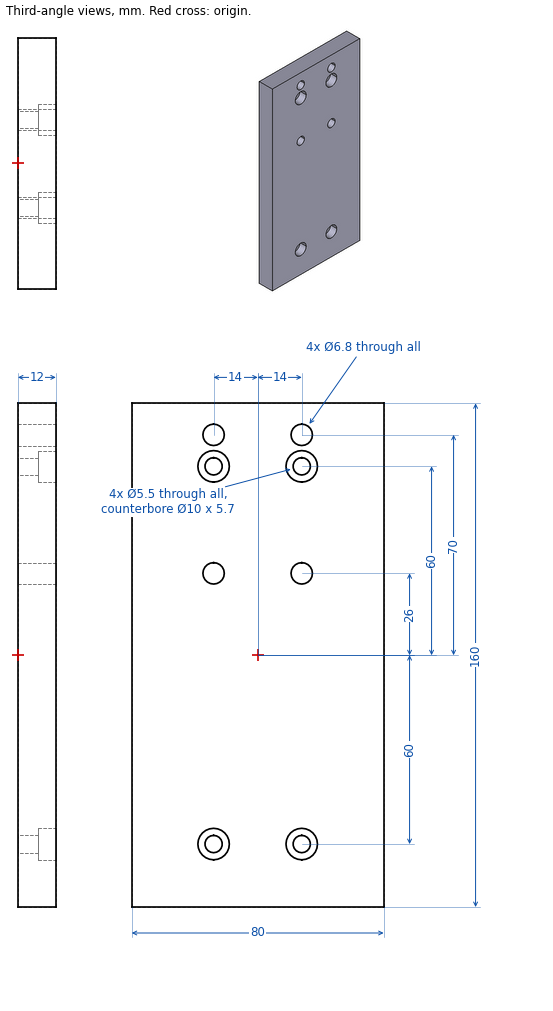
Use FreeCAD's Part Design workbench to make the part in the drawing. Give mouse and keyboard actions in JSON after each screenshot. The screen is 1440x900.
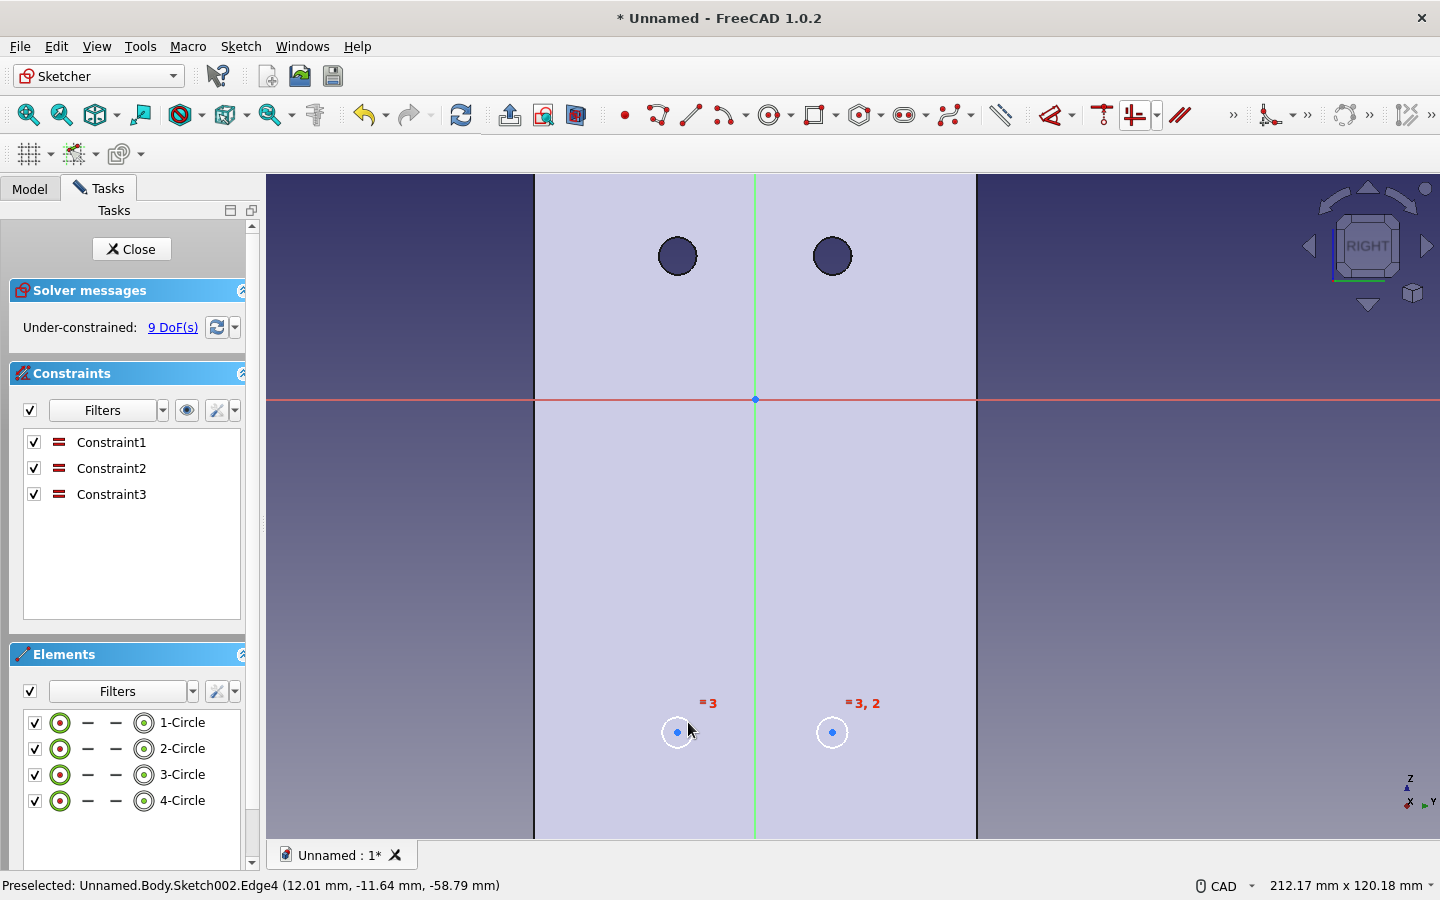
{"action": "scroll", "coordinate": [844, 723], "scroll_direction": "down", "scroll_amount": 2}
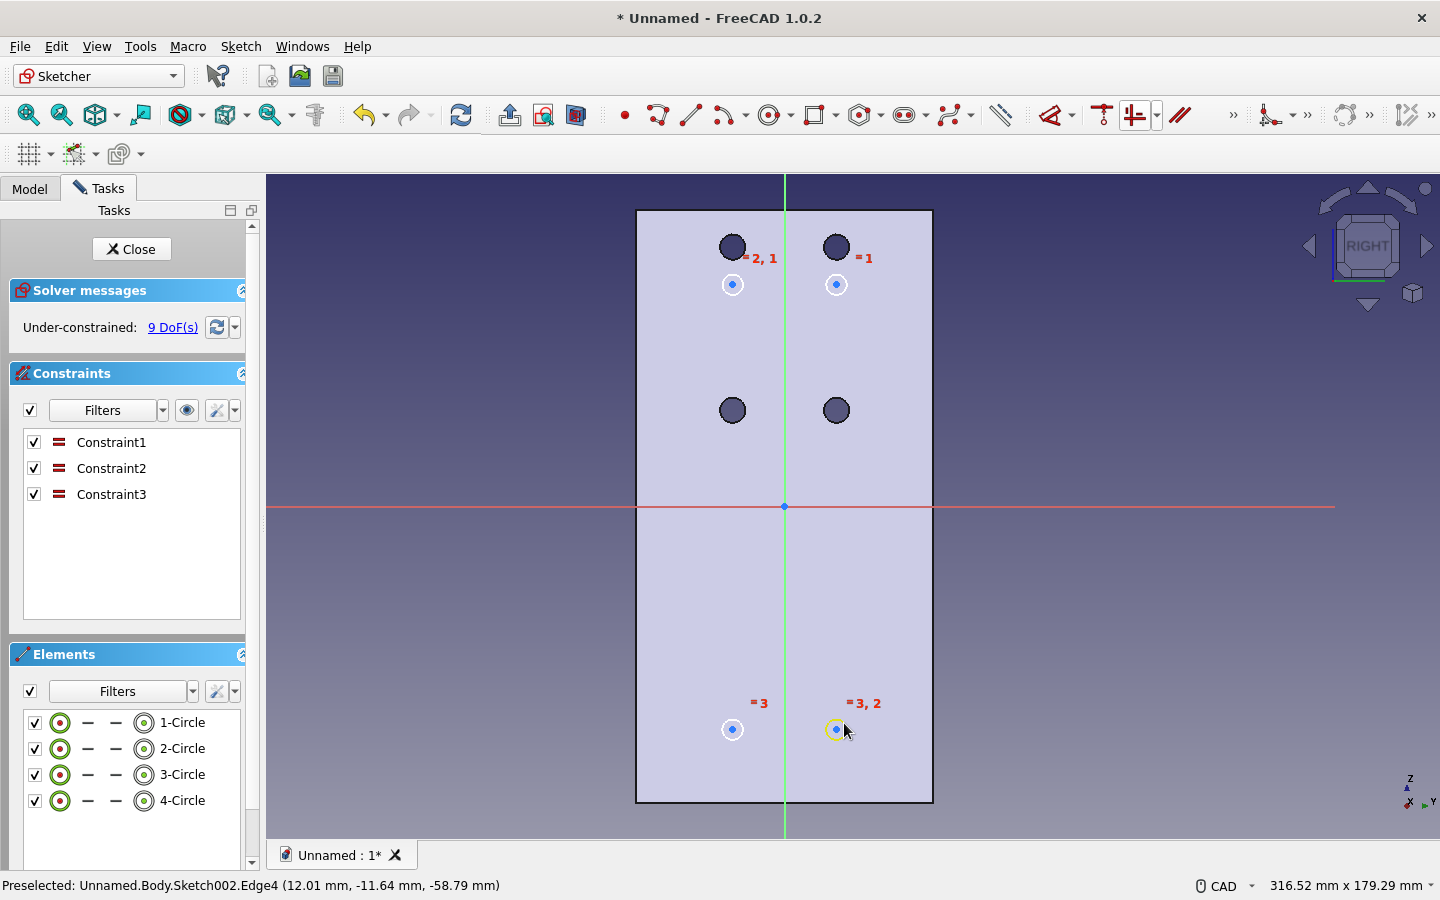
{"action": "left_click", "coordinate": [837, 285]}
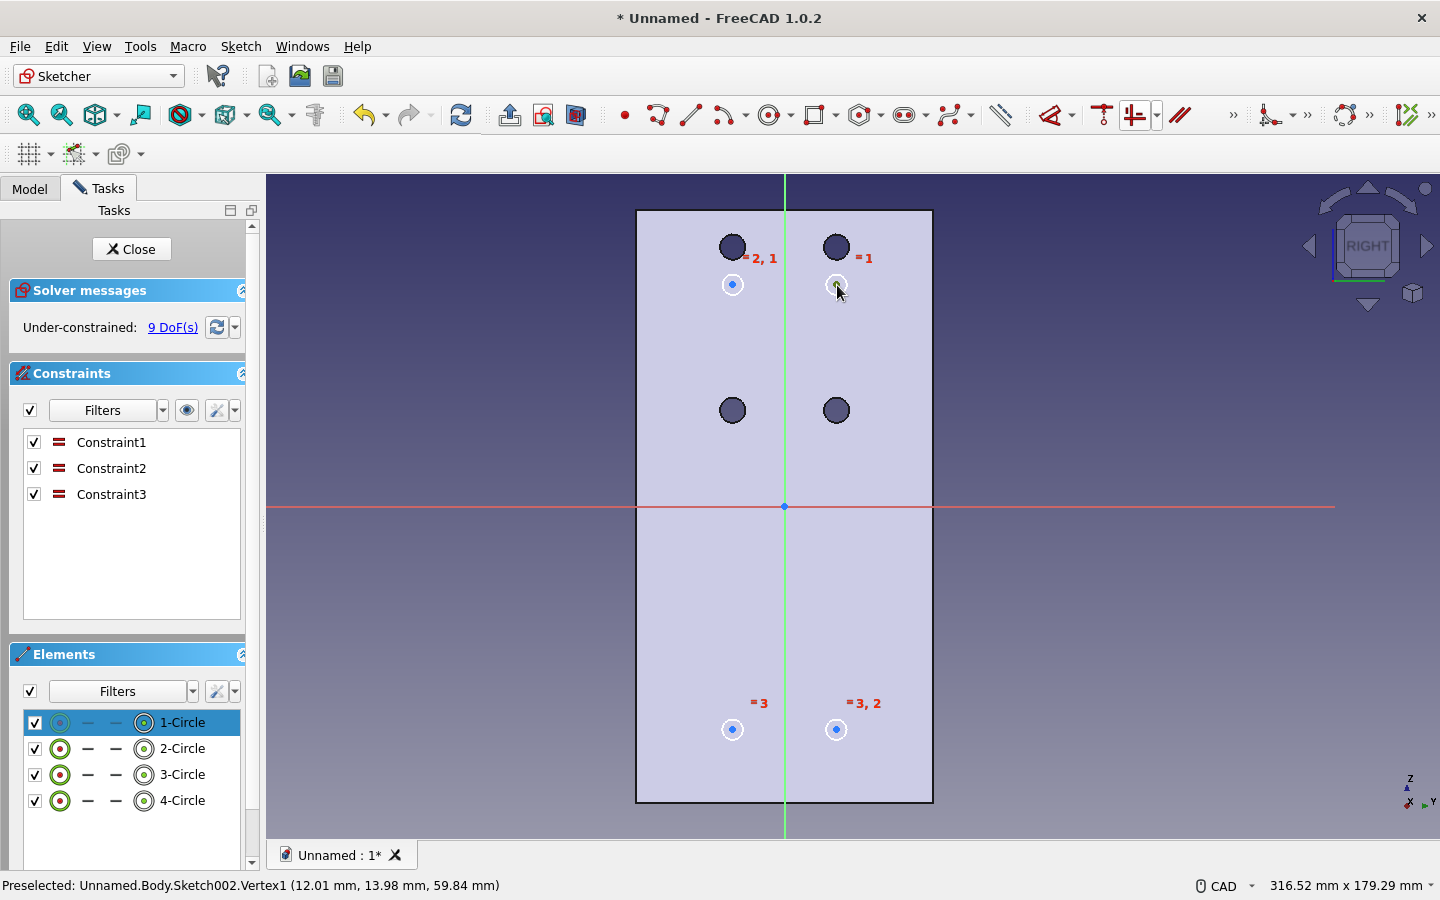
{"action": "left_click", "coordinate": [733, 285]}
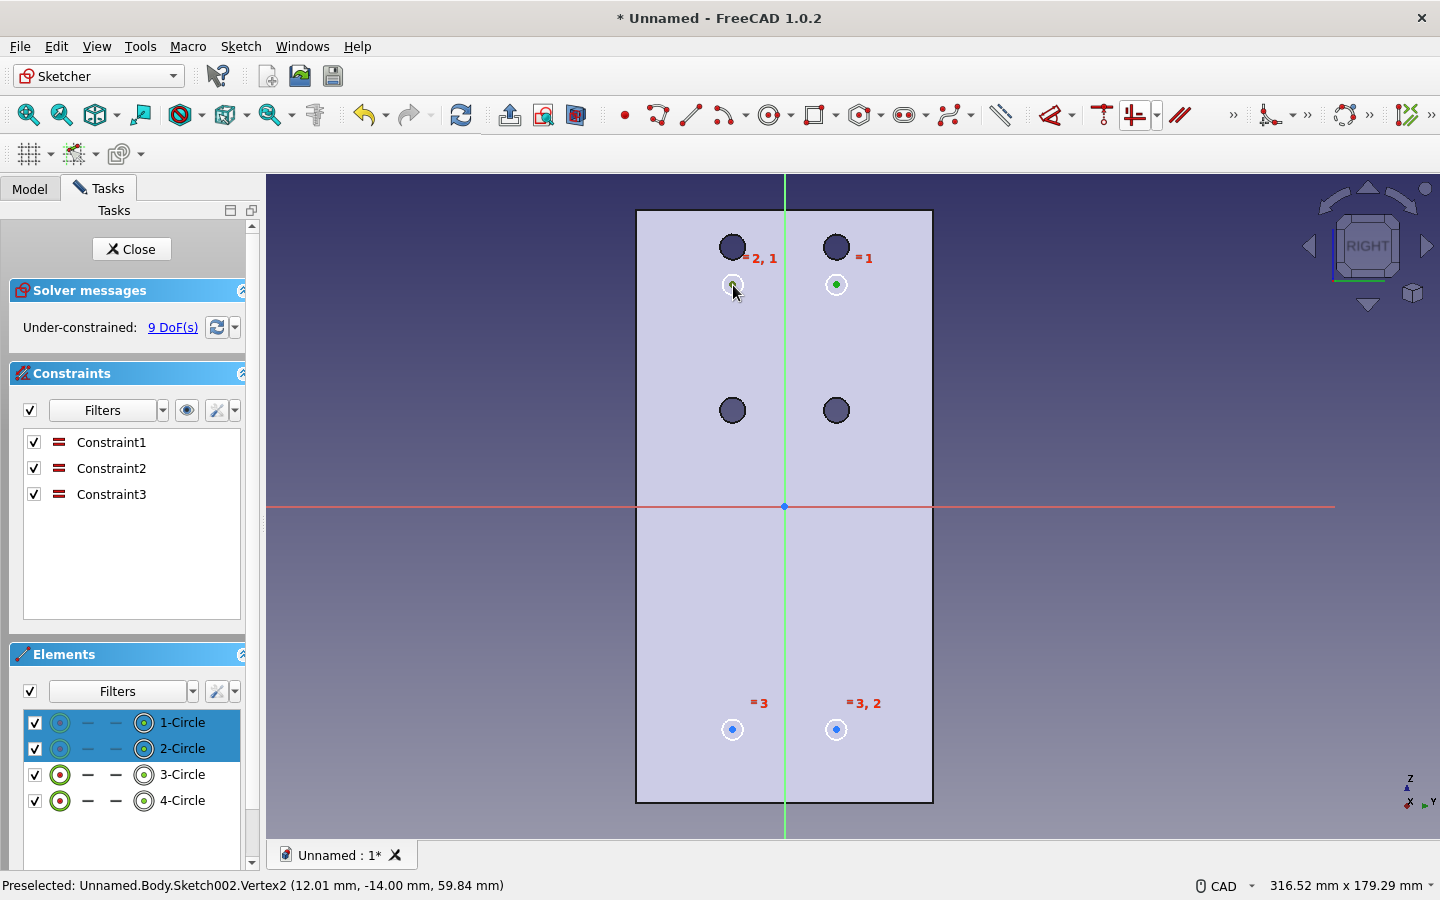
{"action": "left_click", "coordinate": [1156, 116]}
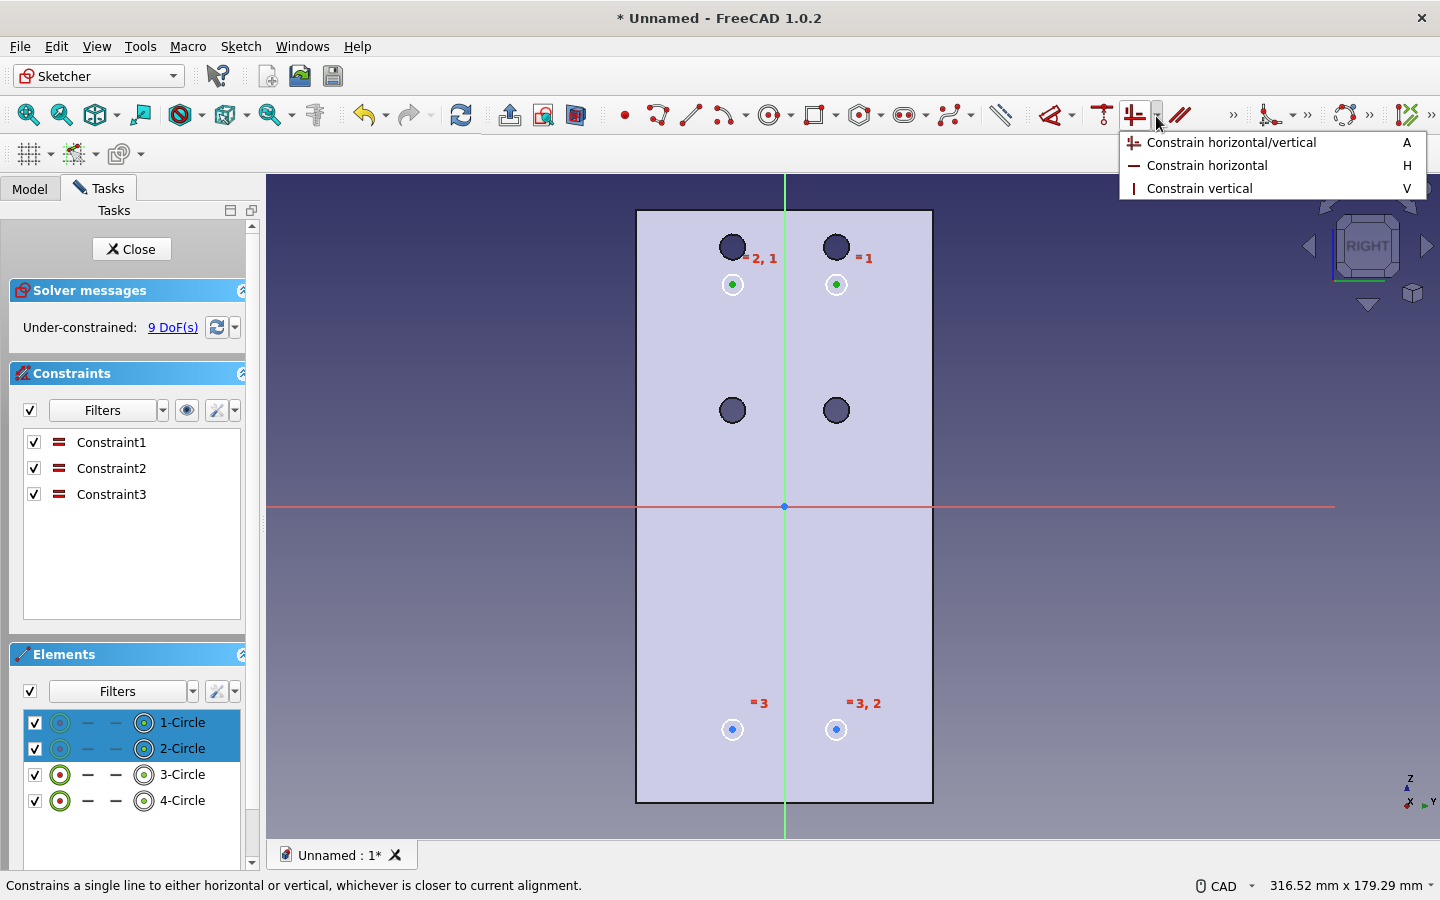
{"action": "left_click", "coordinate": [1273, 166]}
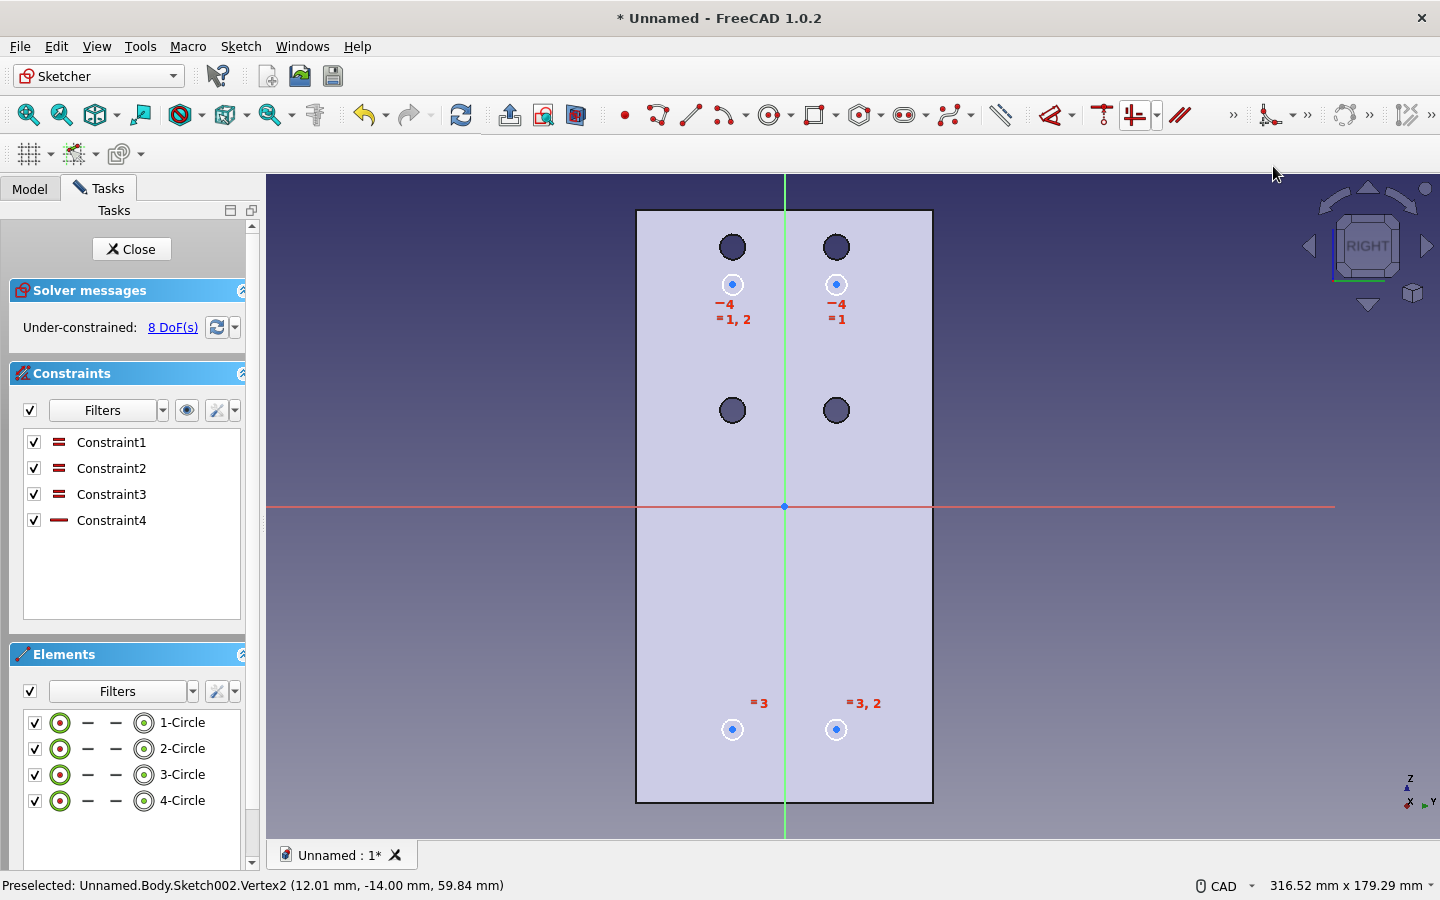
{"action": "left_click", "coordinate": [837, 285]}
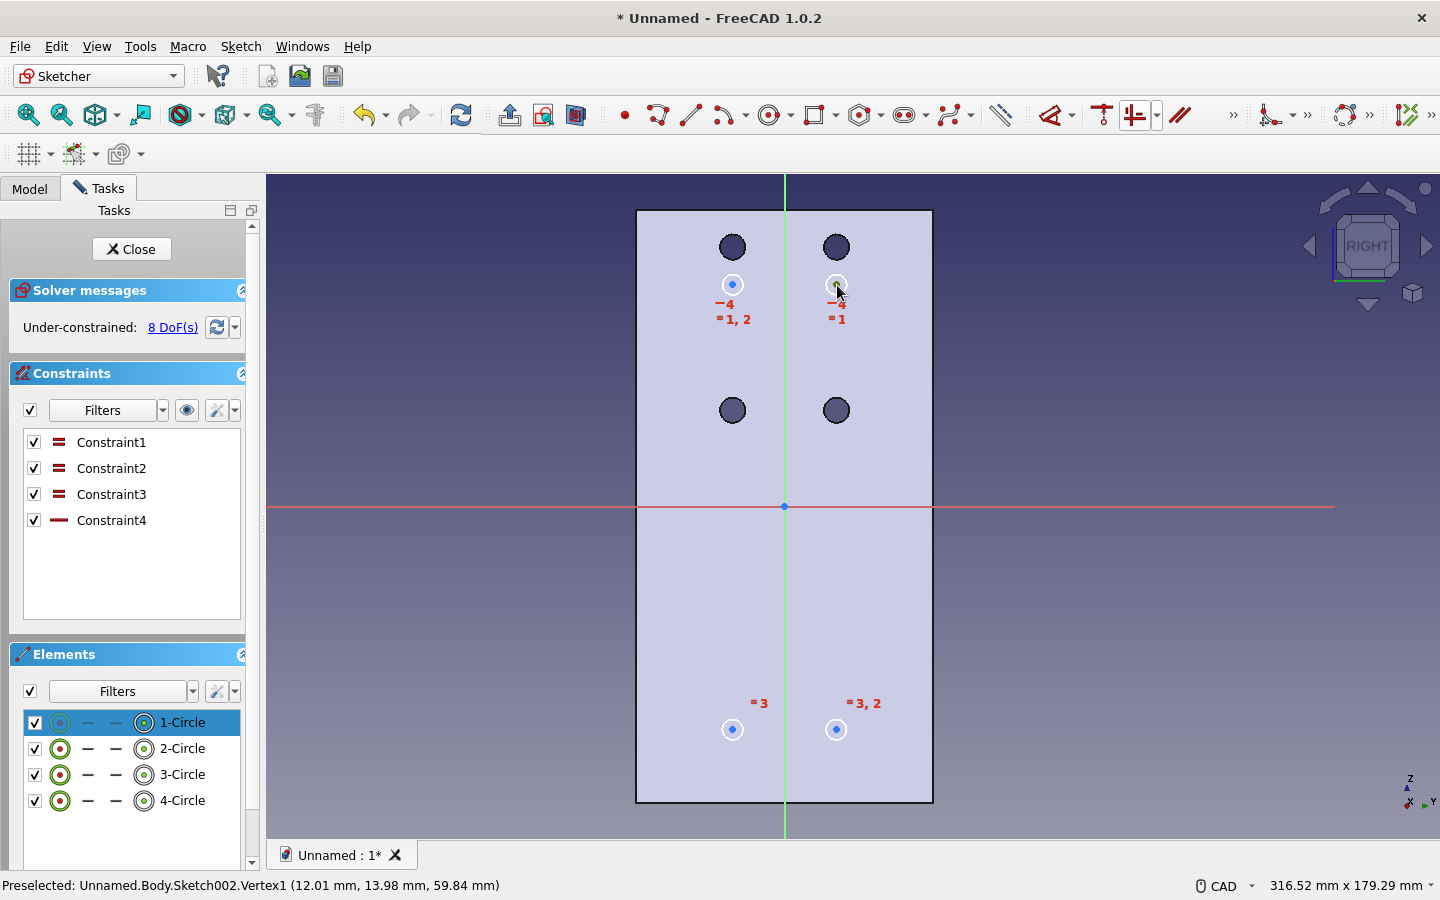
{"action": "left_click", "coordinate": [836, 730]}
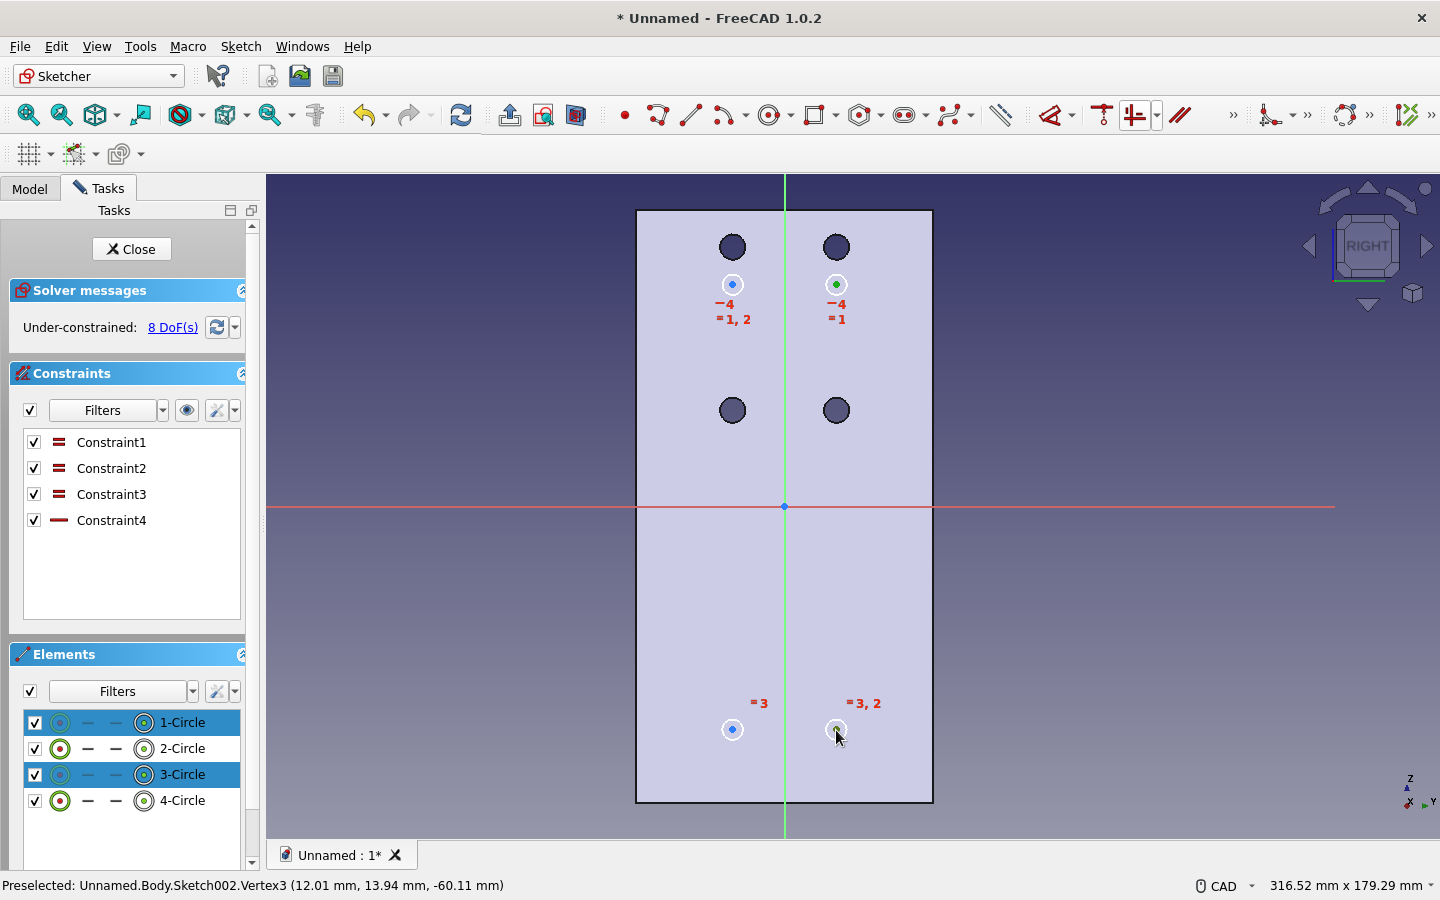
{"action": "key", "text": "v"}